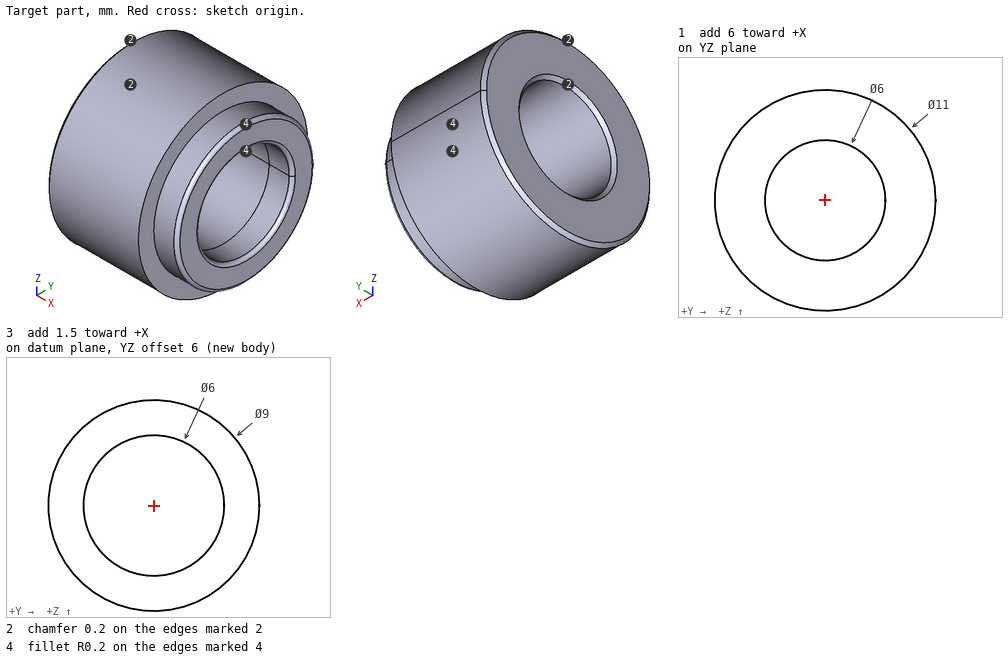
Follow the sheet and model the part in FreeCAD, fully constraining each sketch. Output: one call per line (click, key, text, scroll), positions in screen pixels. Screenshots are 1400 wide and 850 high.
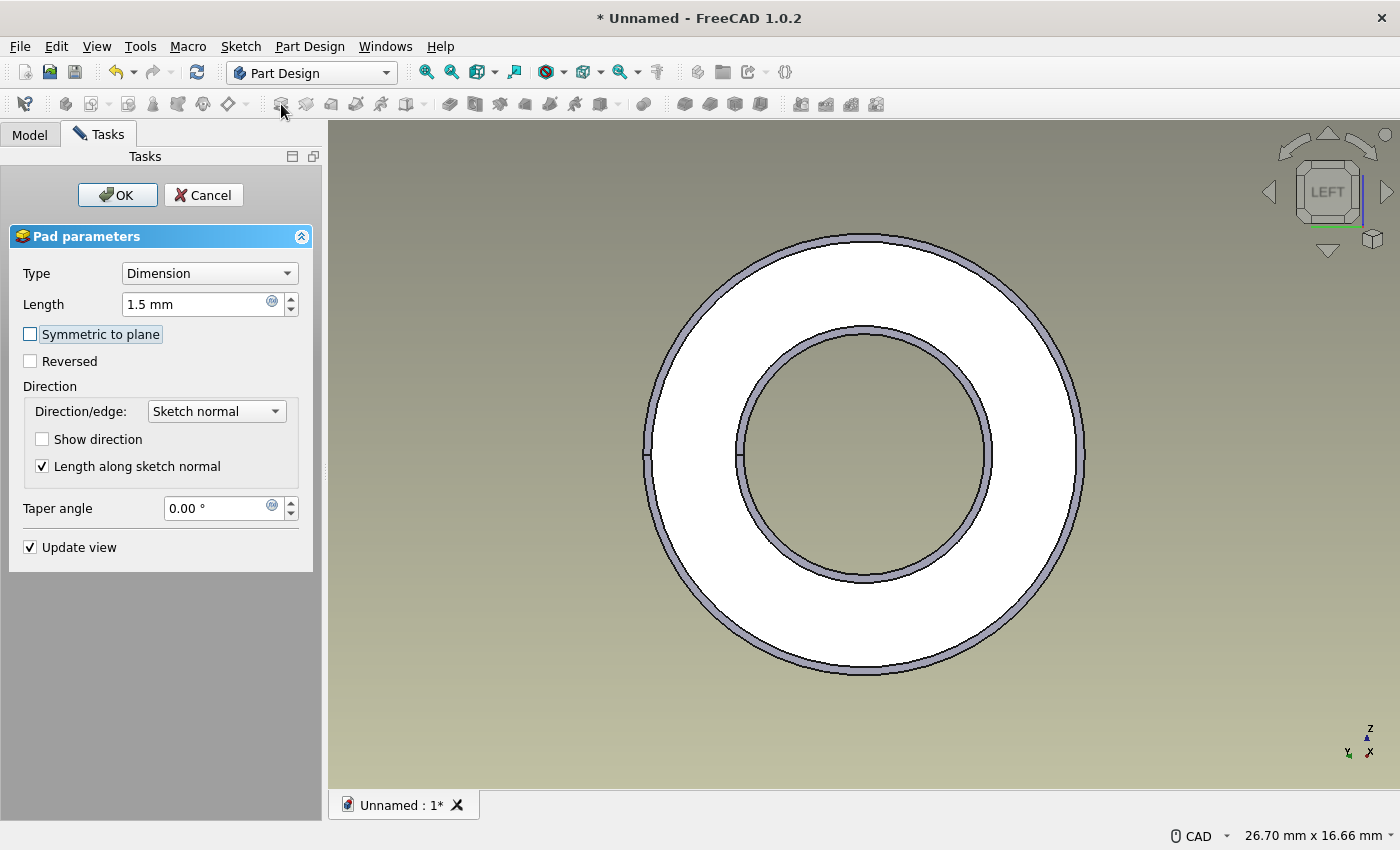
click(118, 195)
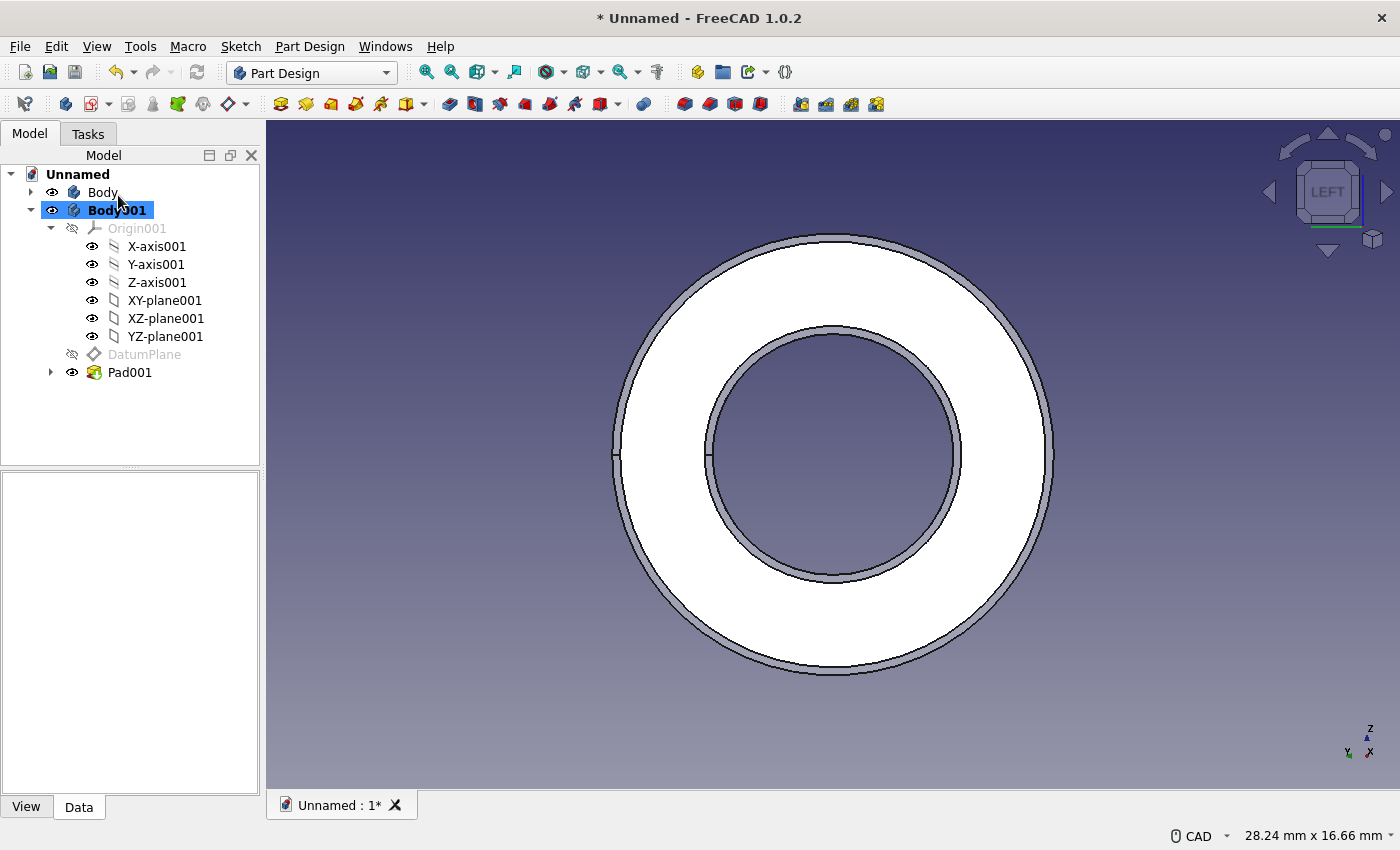
key(0)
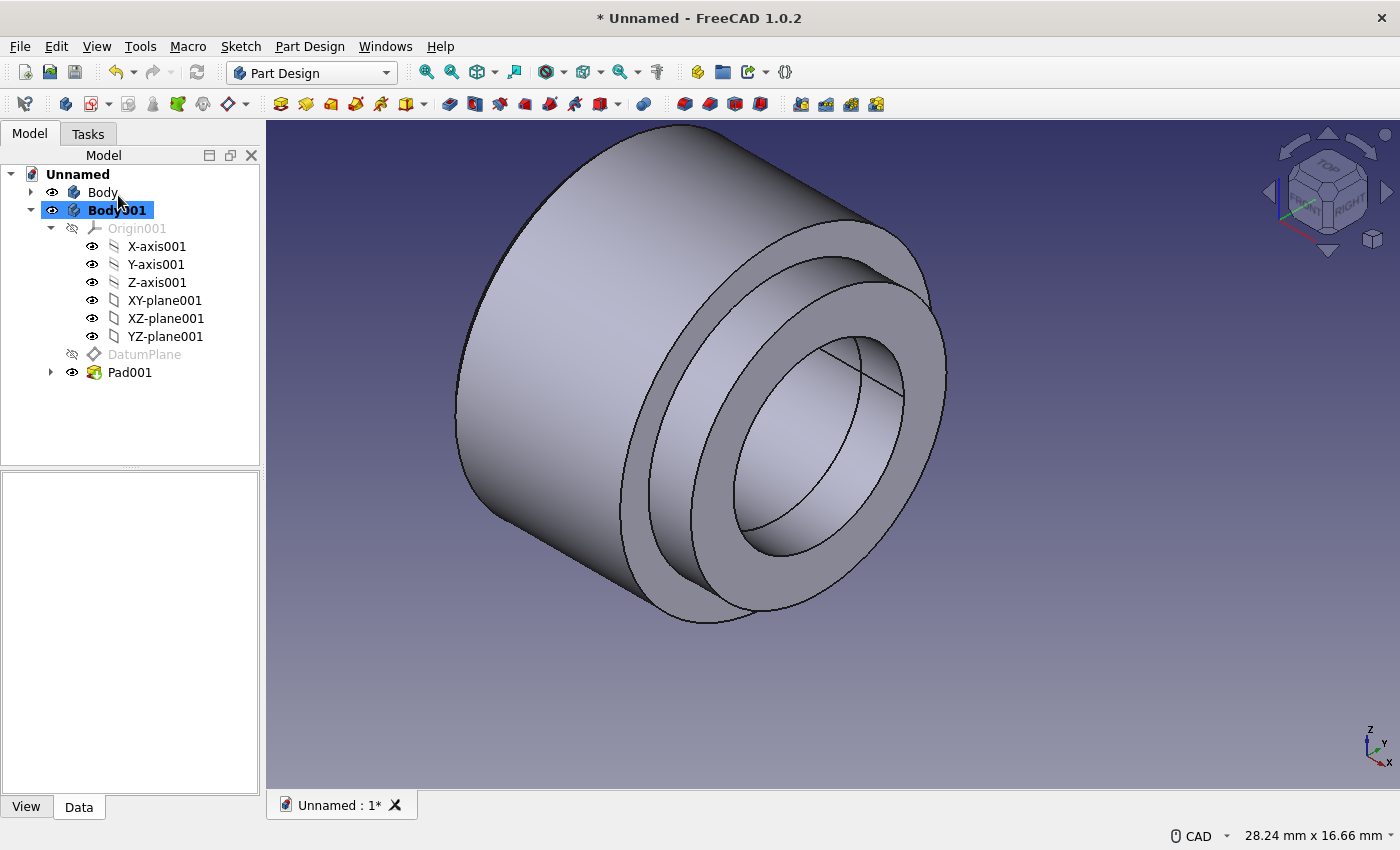
click(691, 519)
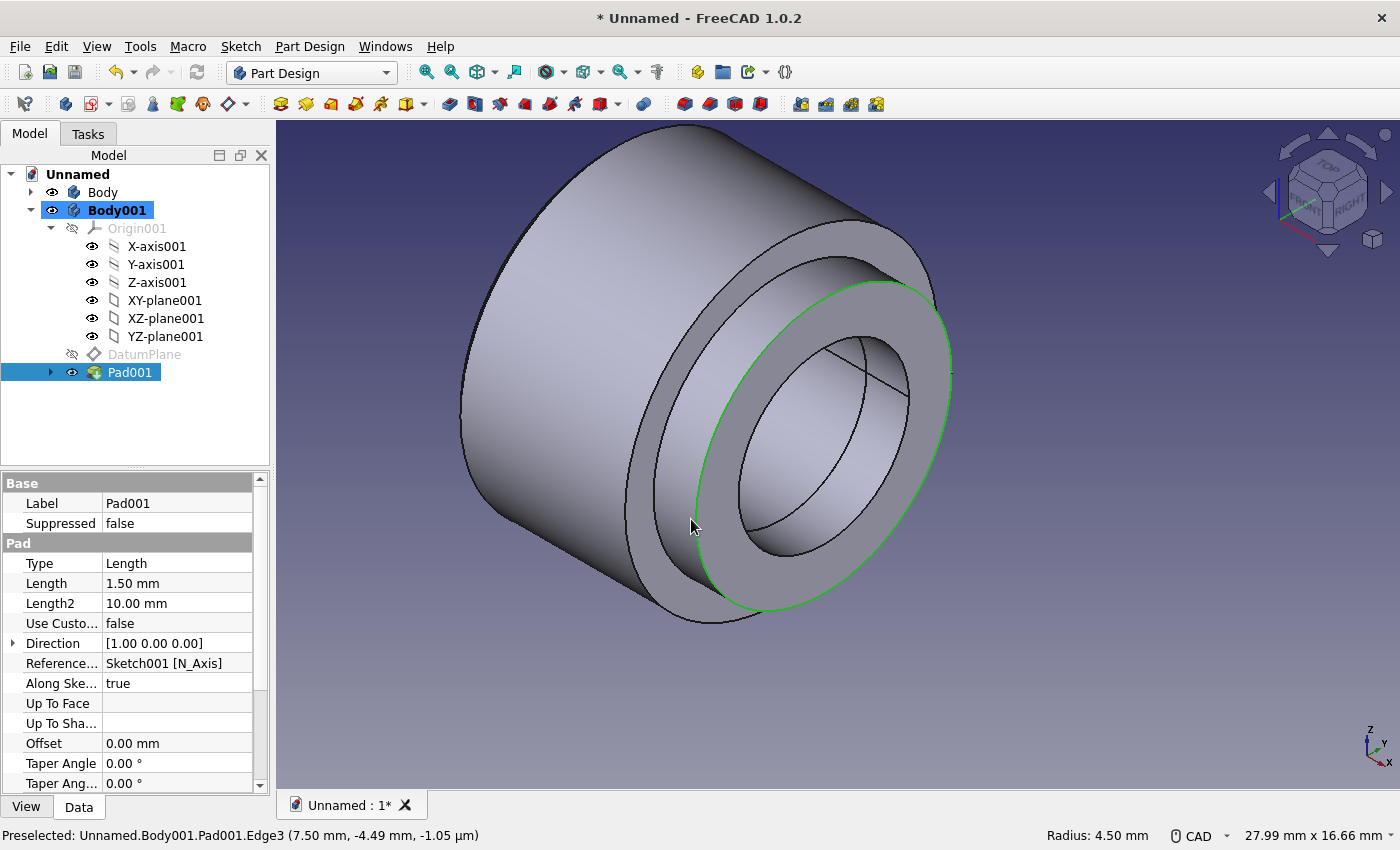
click(797, 554, ctrl)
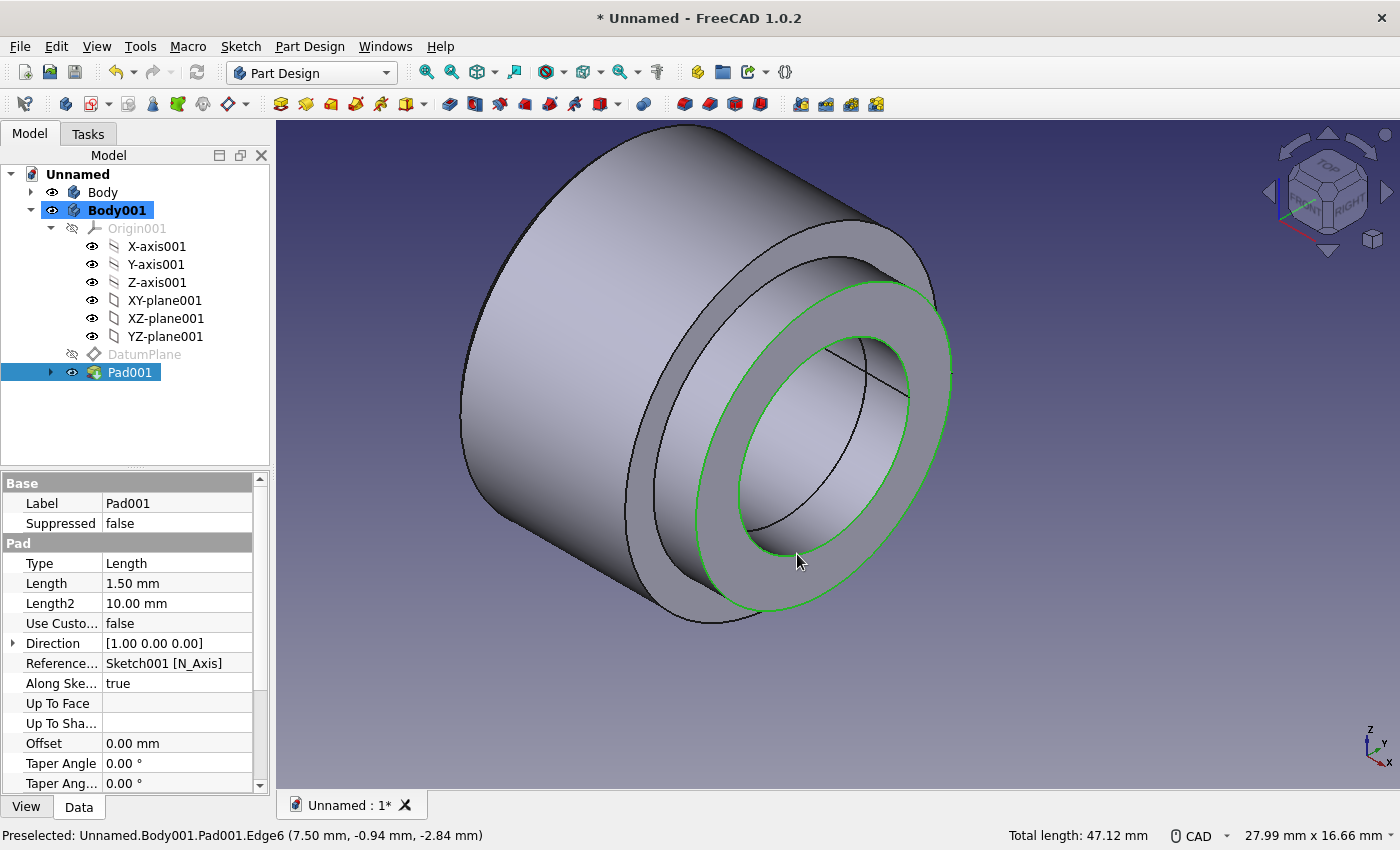
click(685, 104)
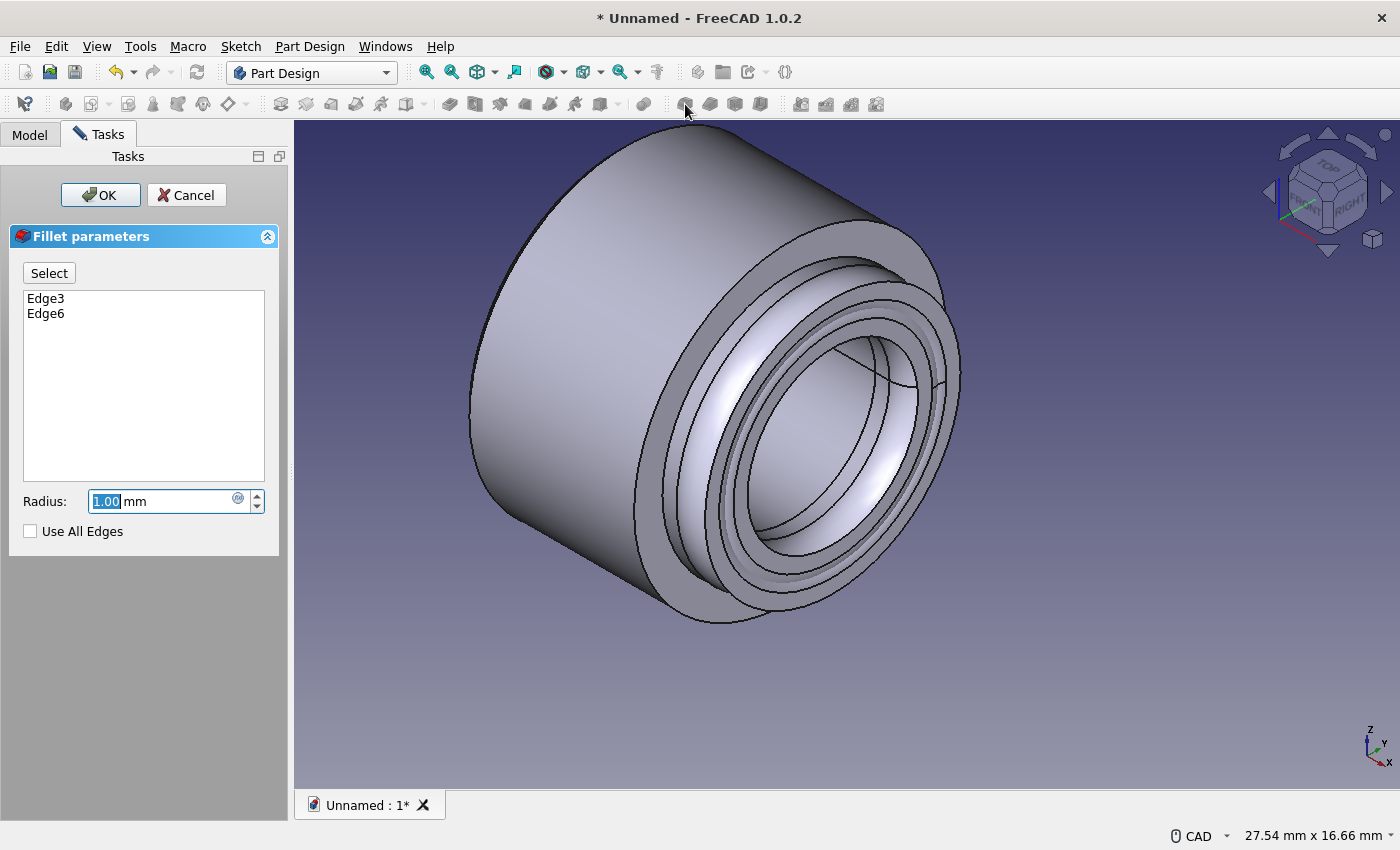
text(0.2)
key(Tab)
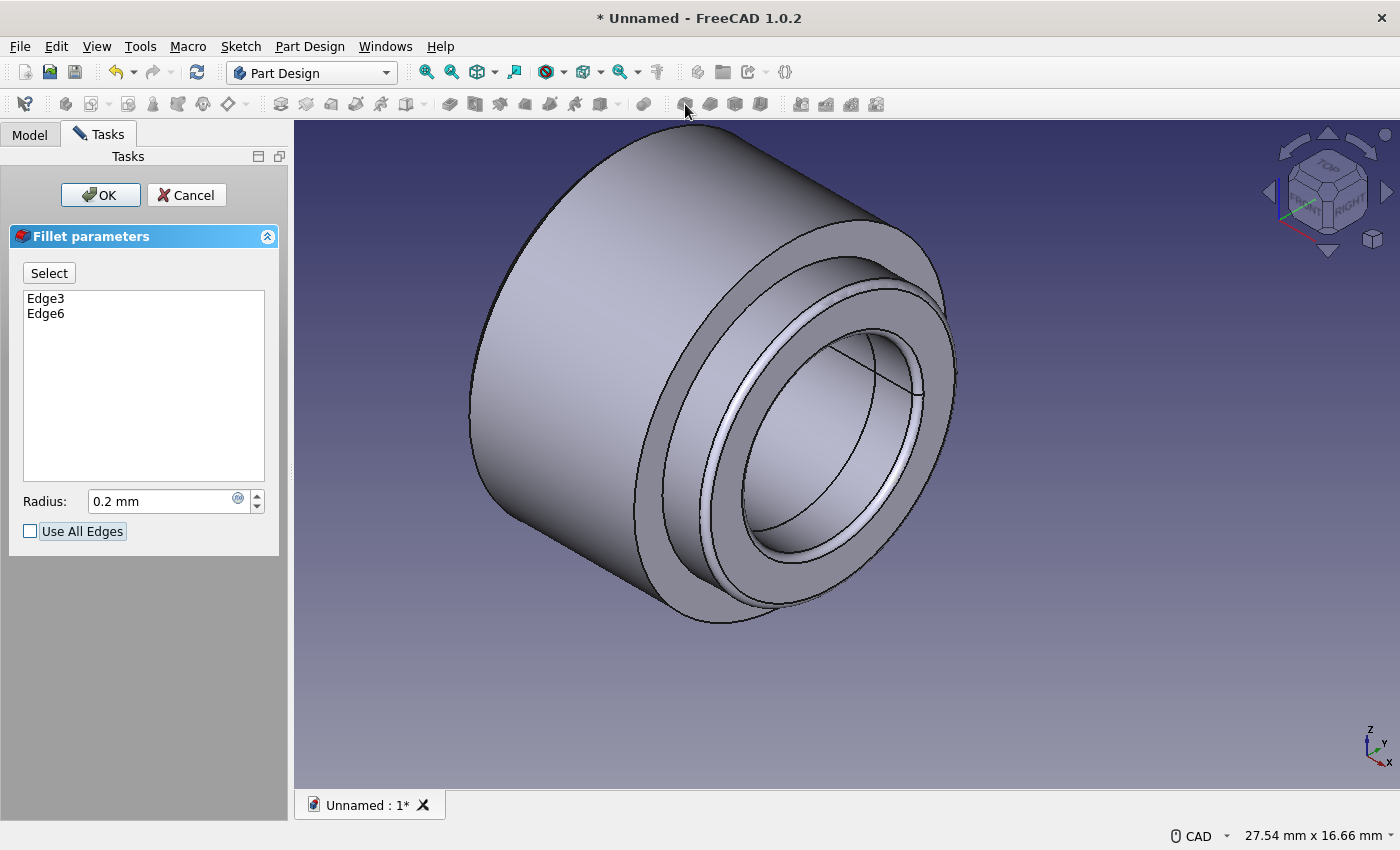
click(101, 195)